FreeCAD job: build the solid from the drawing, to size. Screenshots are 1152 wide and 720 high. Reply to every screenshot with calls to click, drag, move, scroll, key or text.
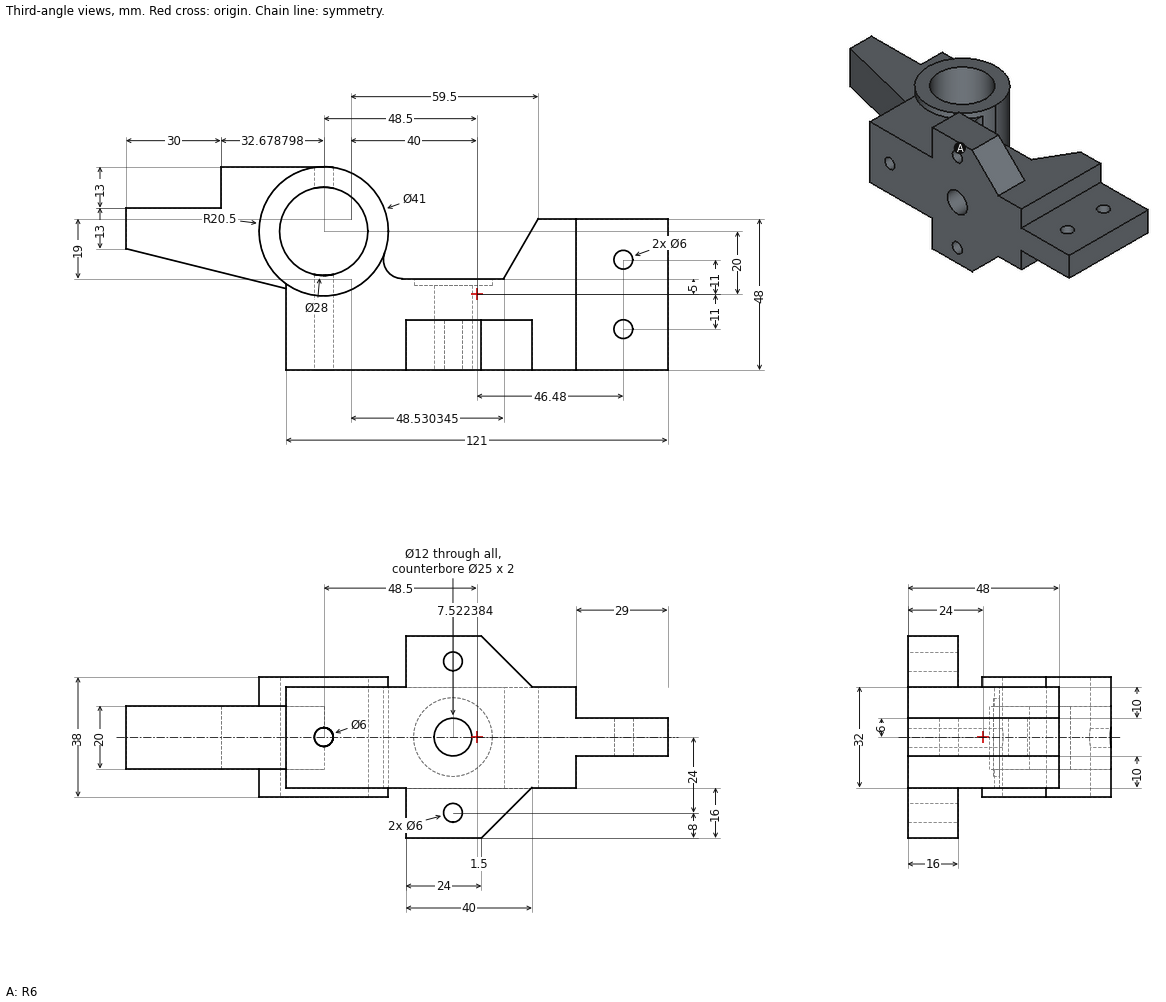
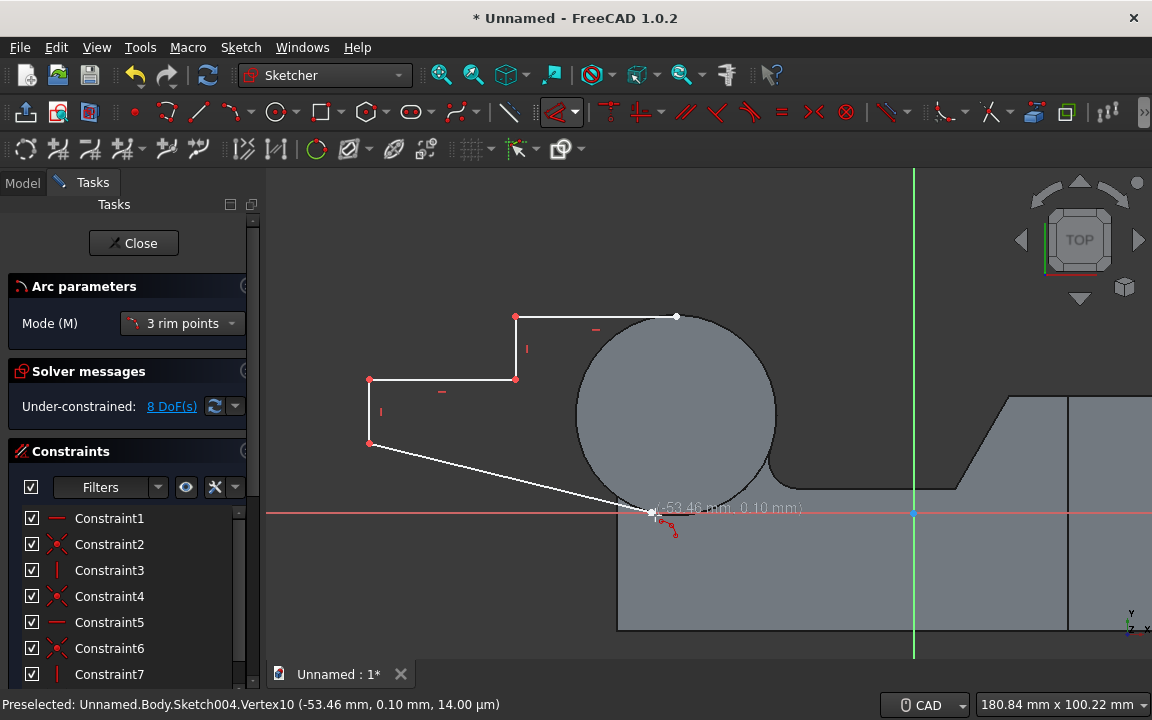
click(677, 317)
click(576, 403)
key(Escape)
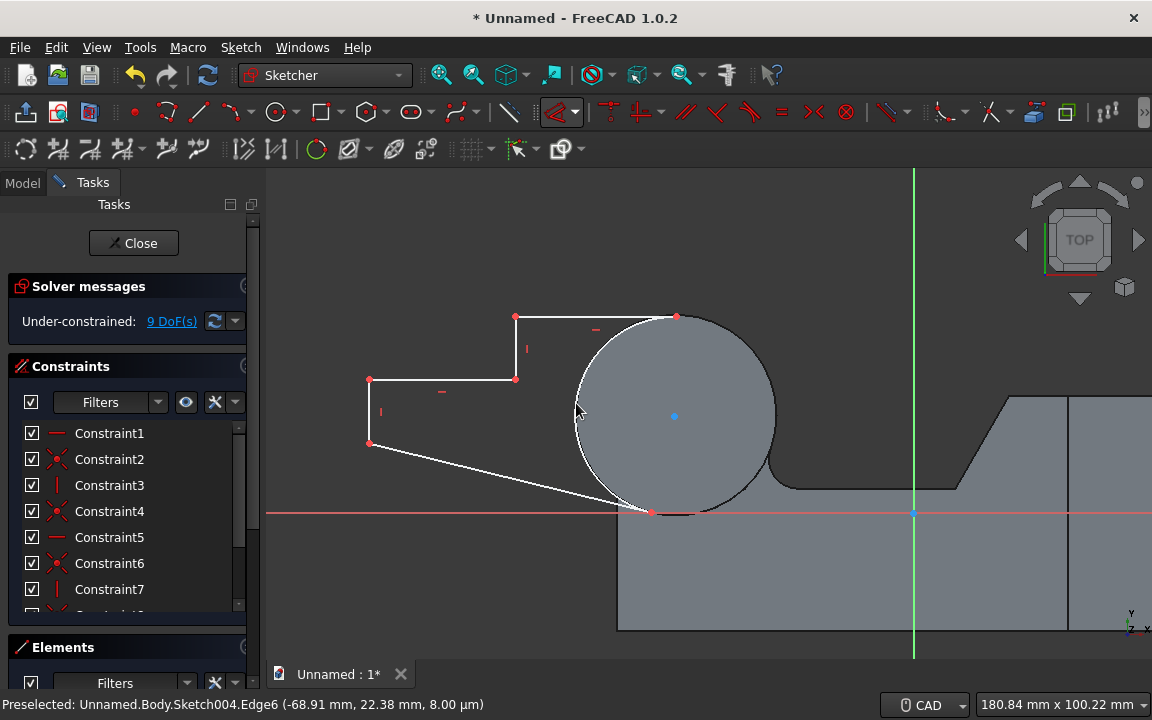
scroll(628, 317, up, 2)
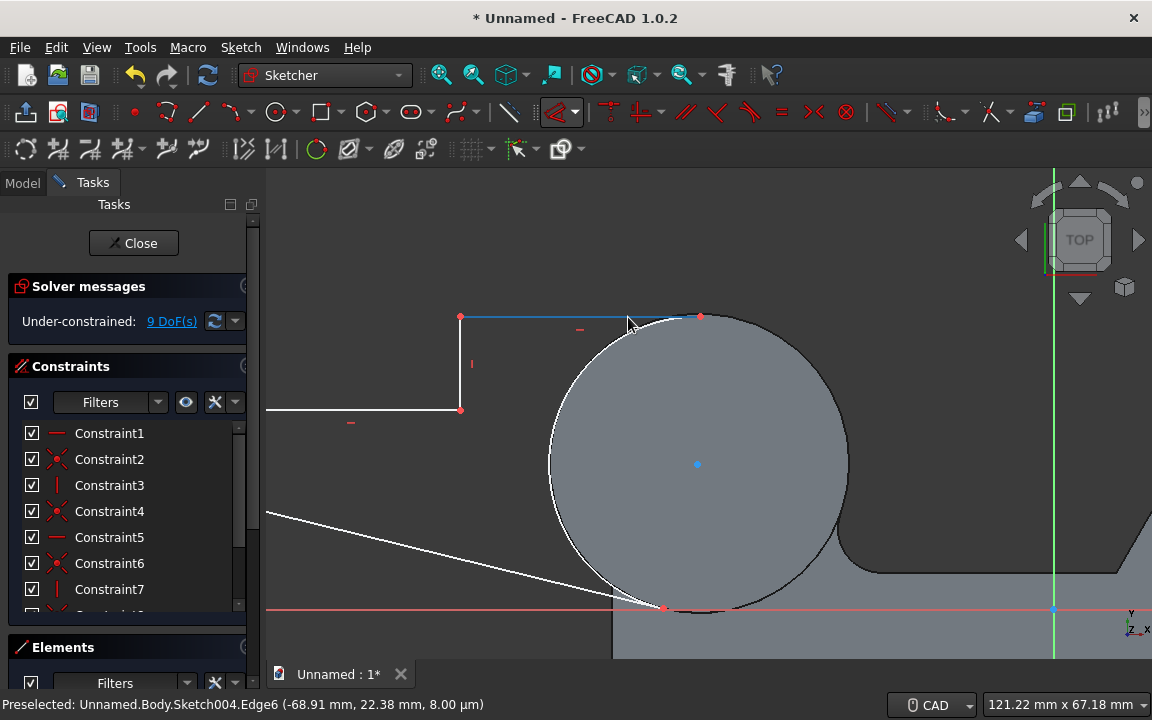
click(628, 317)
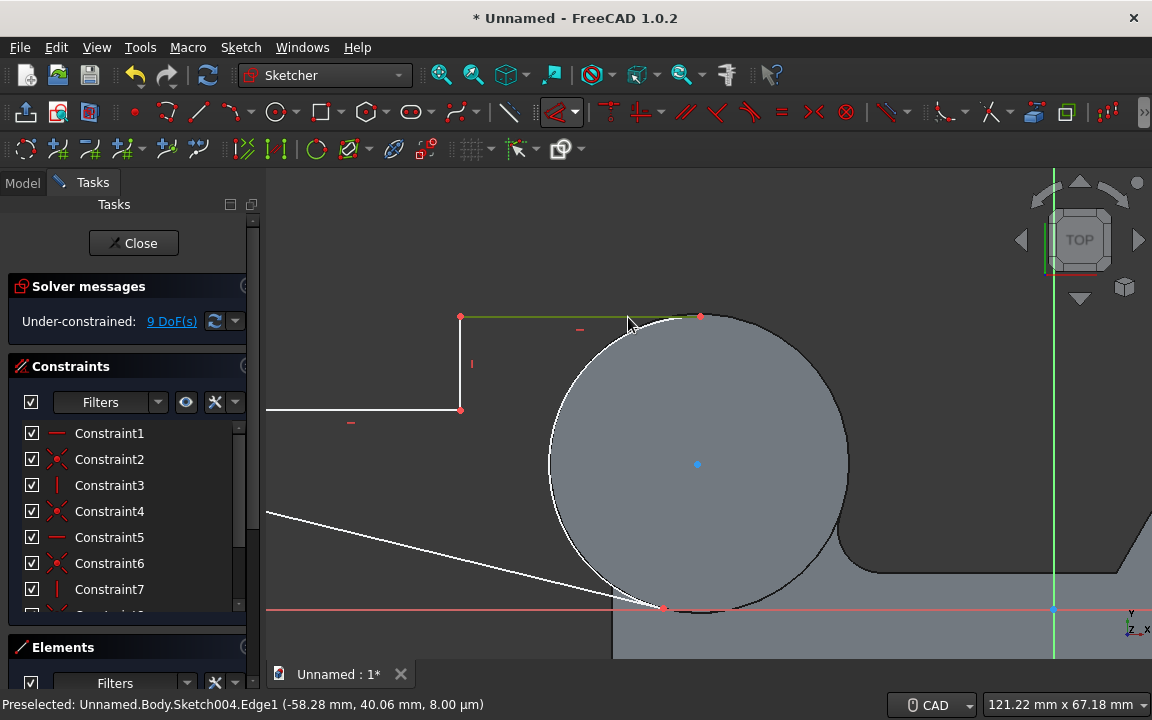
click(585, 368)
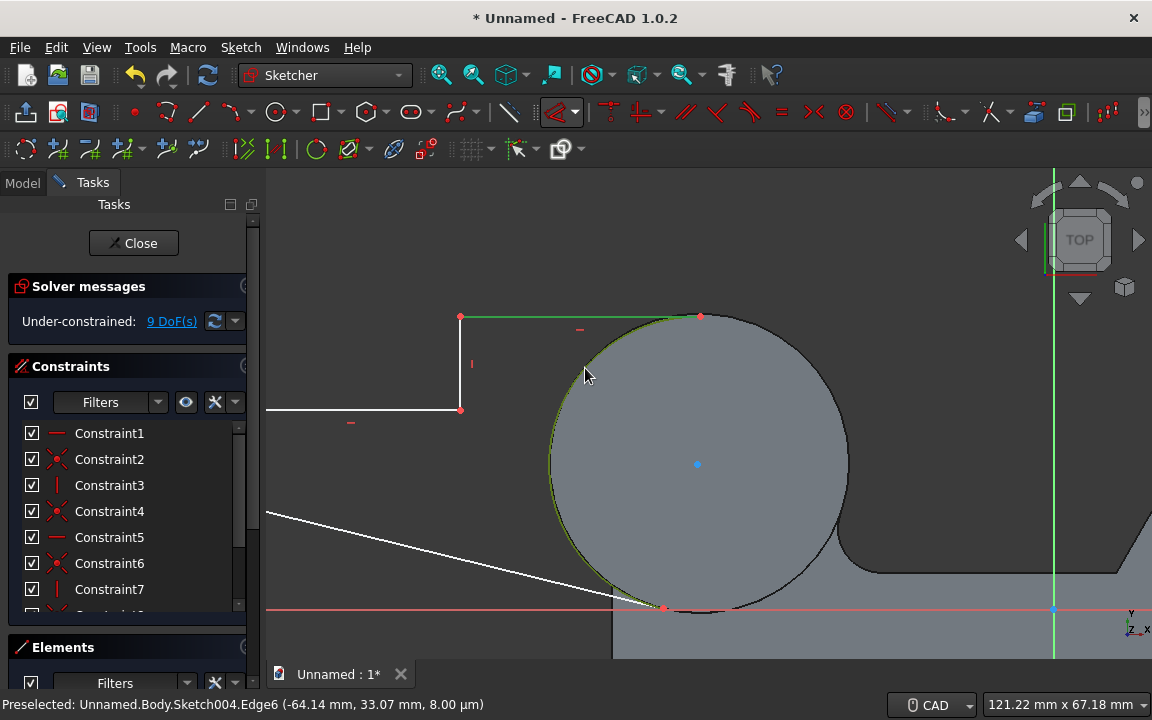
key(t)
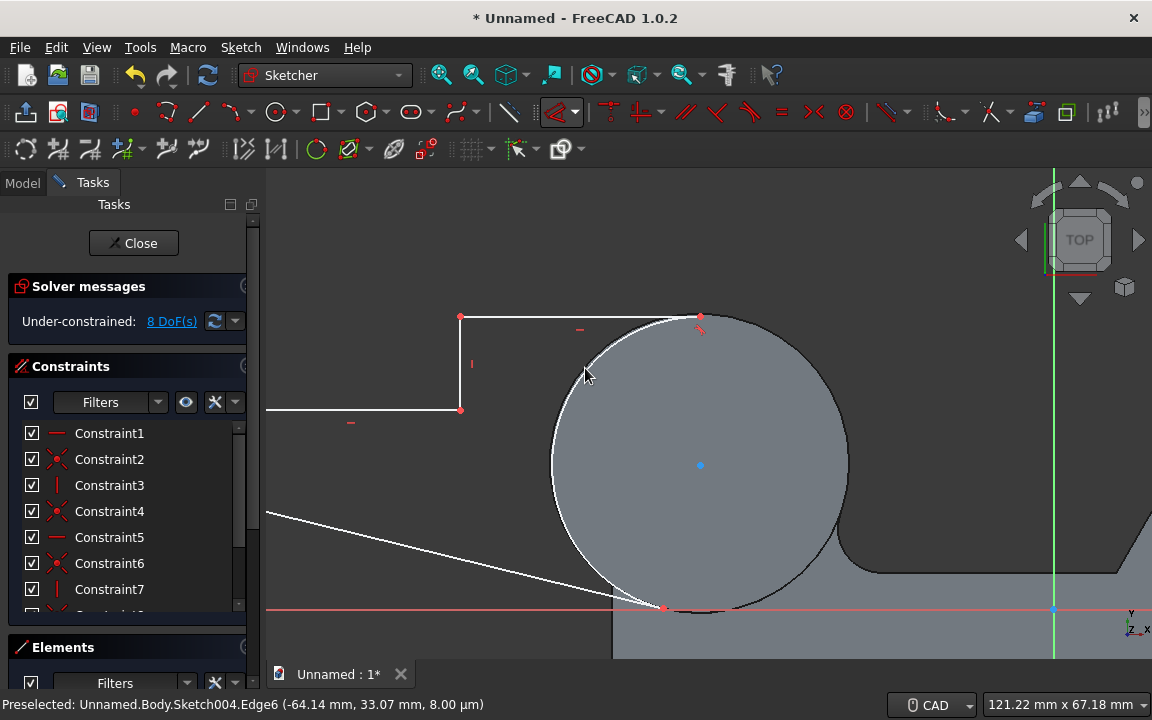
click(368, 537)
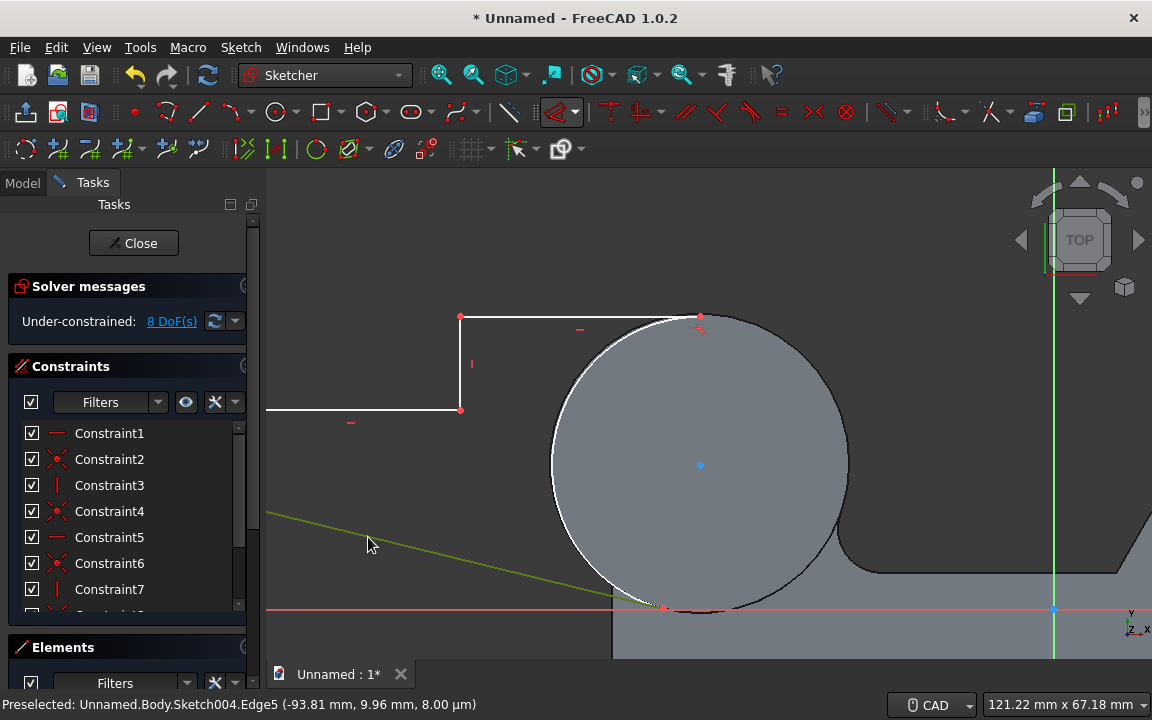
click(587, 369)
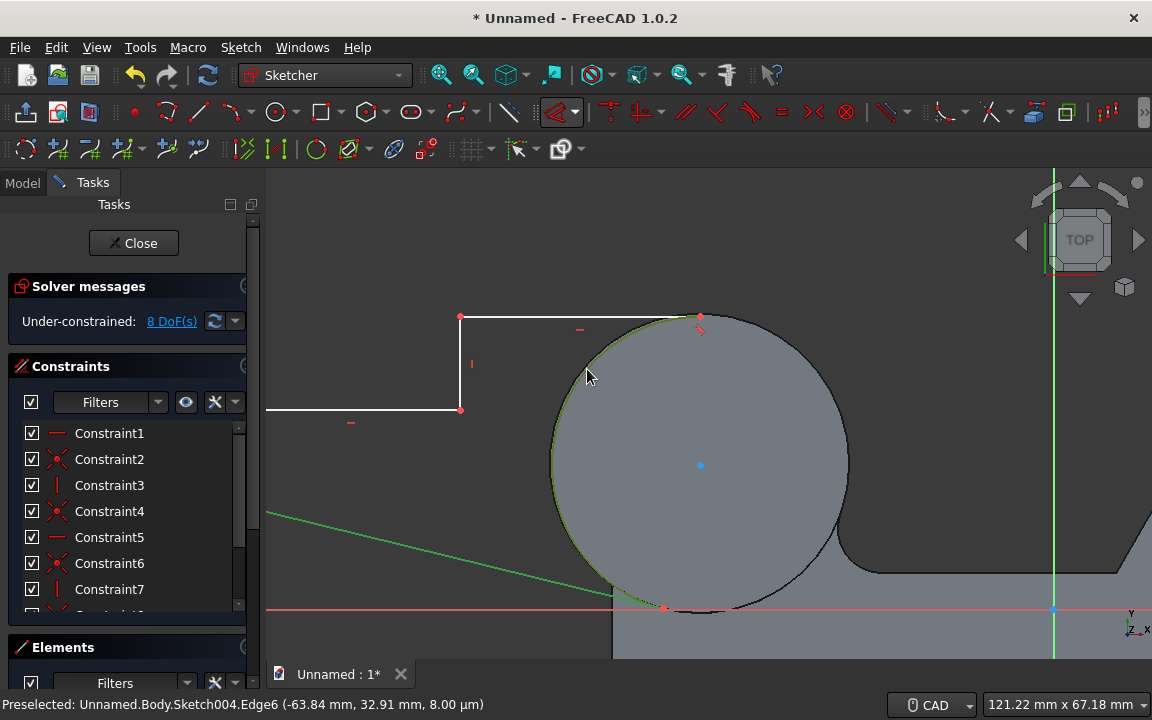
key(t)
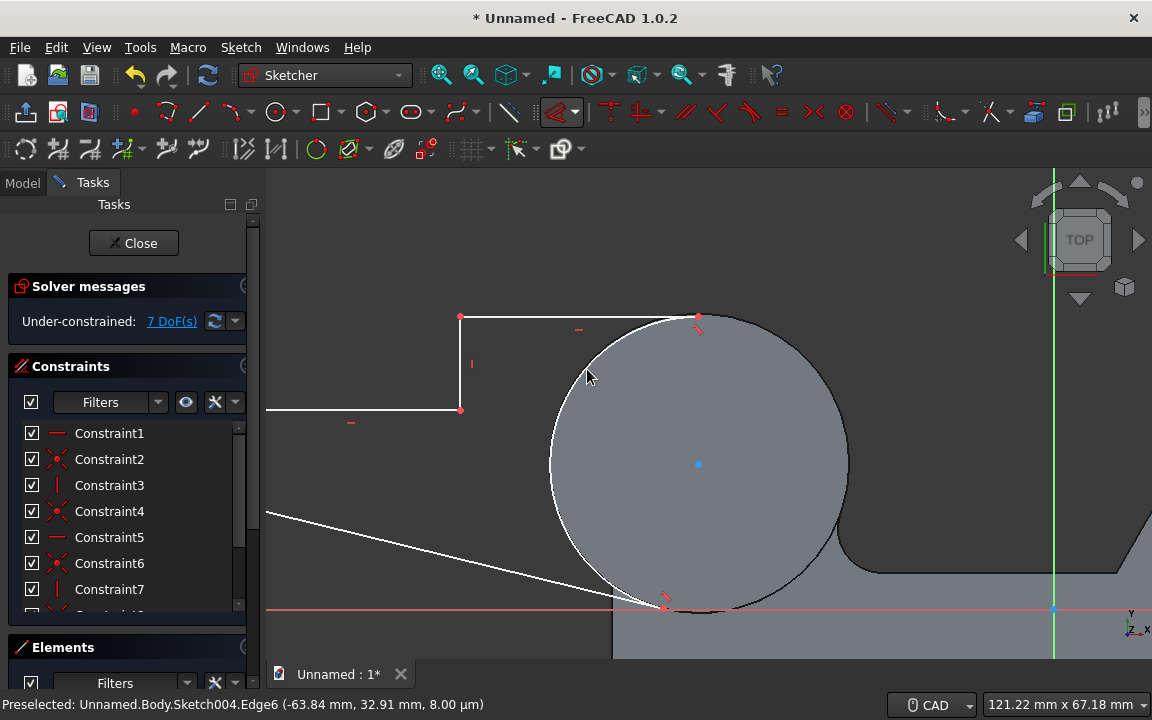
click(585, 369)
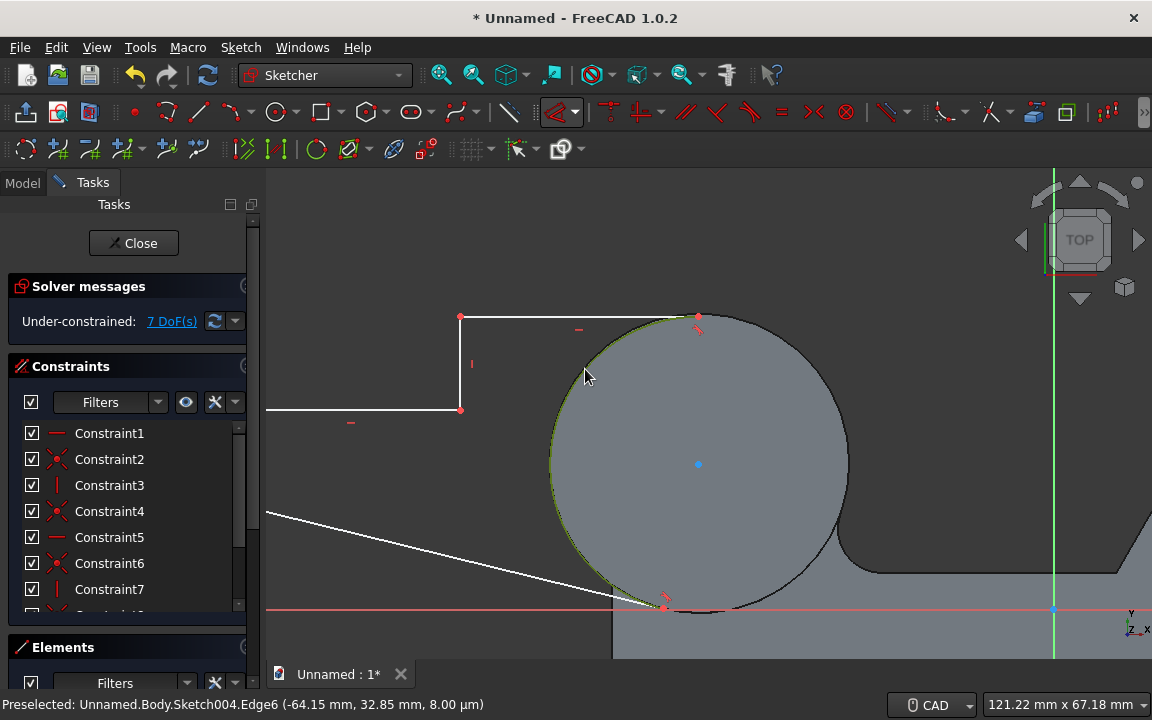
click(578, 112)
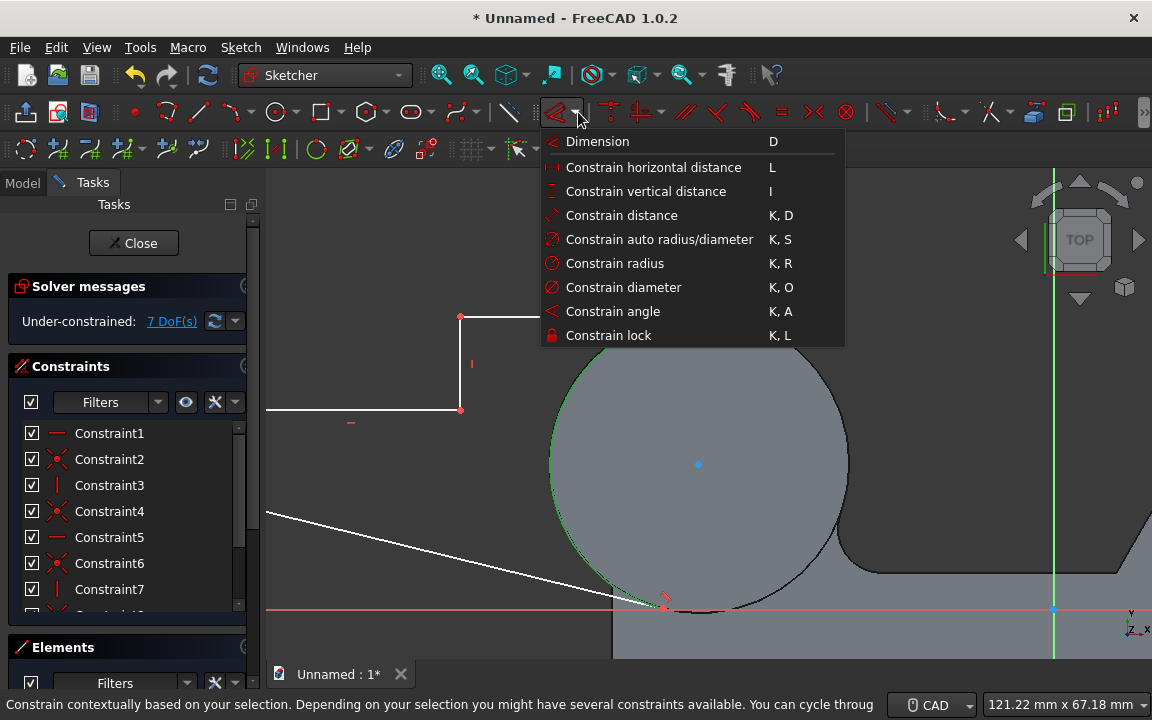
click(693, 263)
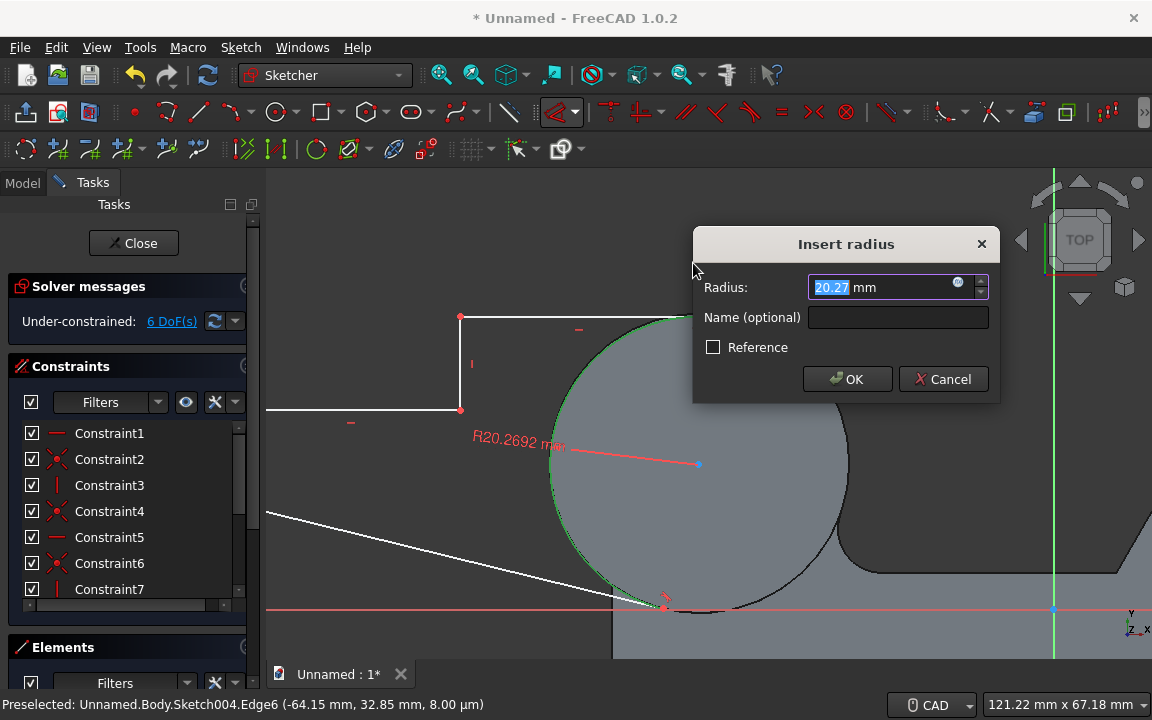
text(20.5)
key(Return)